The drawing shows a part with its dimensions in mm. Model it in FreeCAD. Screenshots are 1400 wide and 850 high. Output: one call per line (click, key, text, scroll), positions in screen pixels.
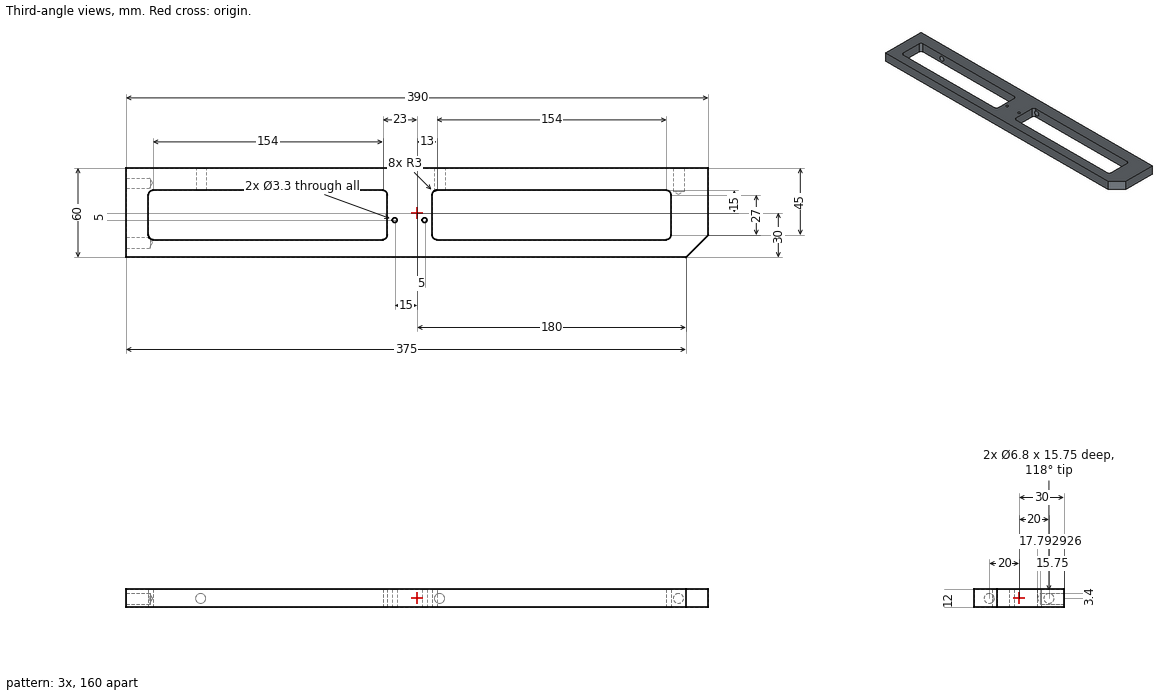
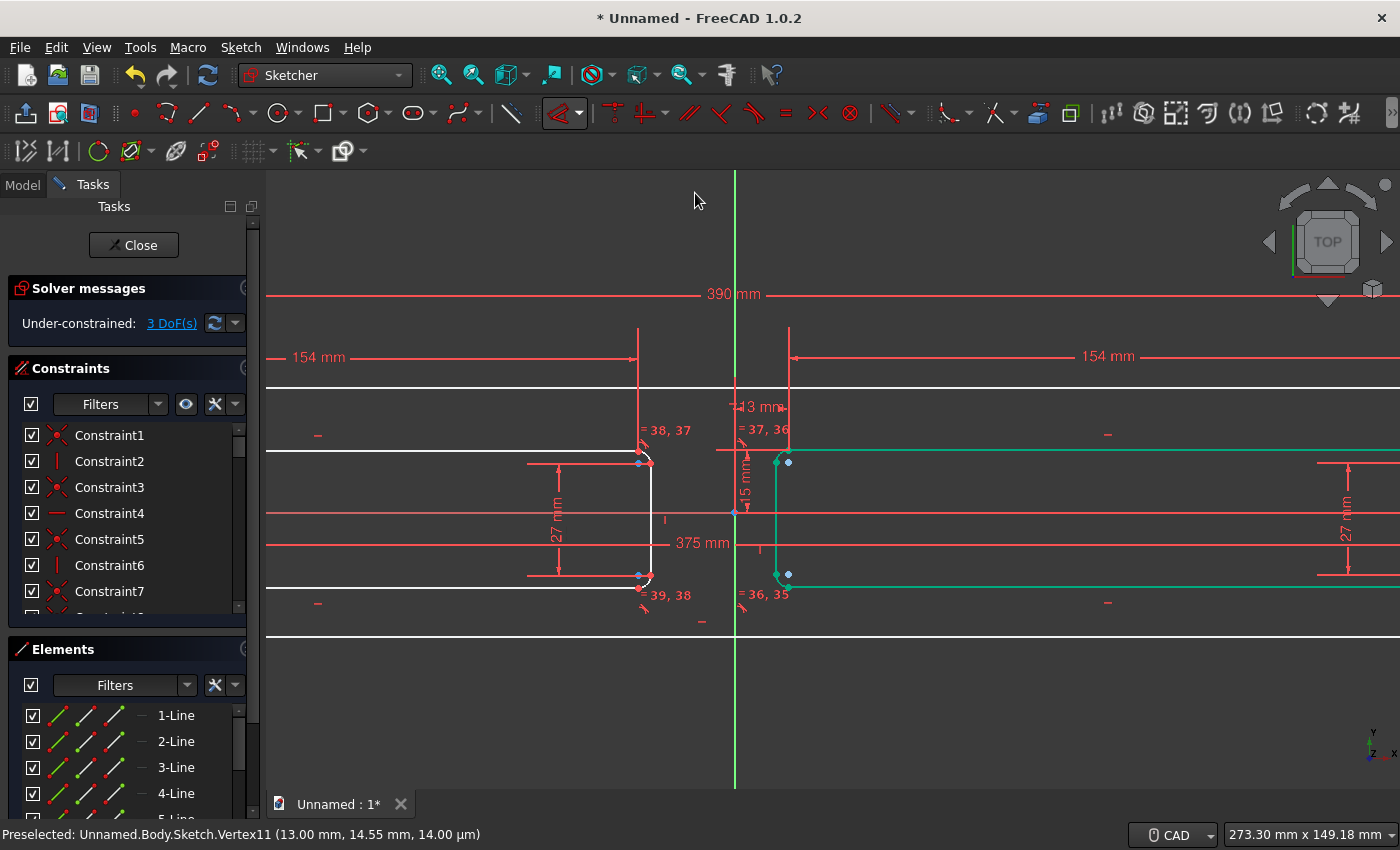
scroll(789, 453, down, 4)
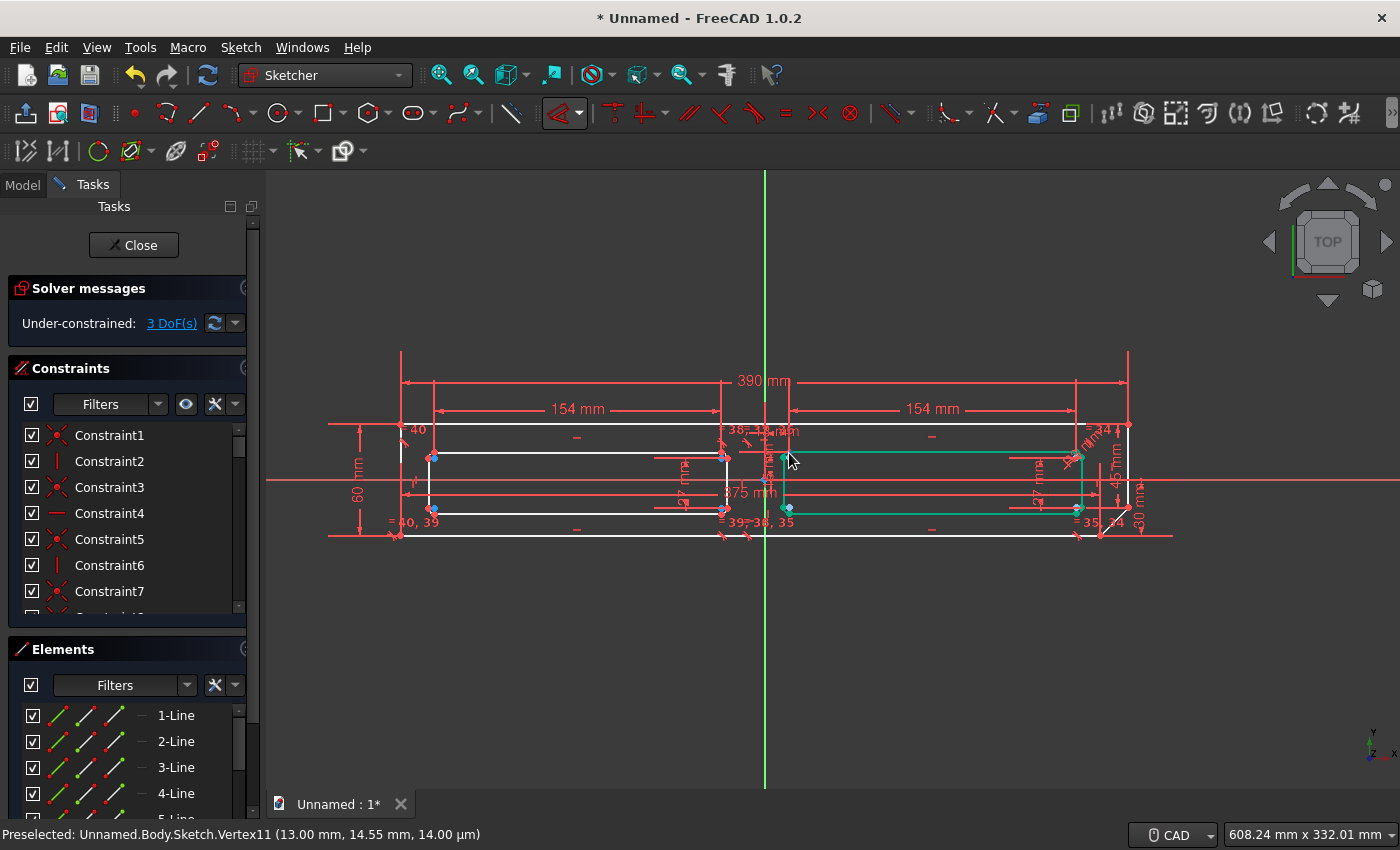
scroll(434, 453, up, 4)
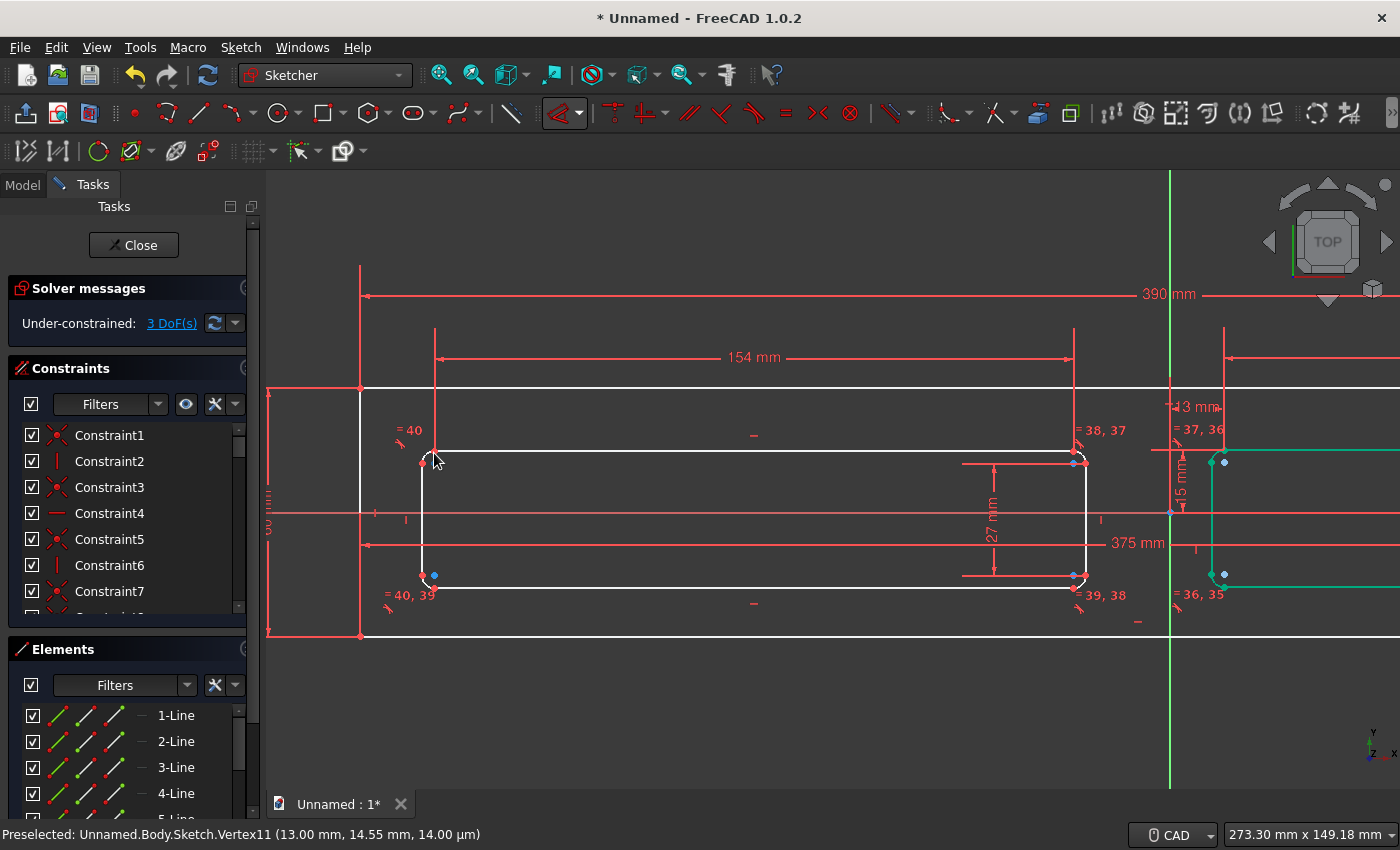
click(435, 451)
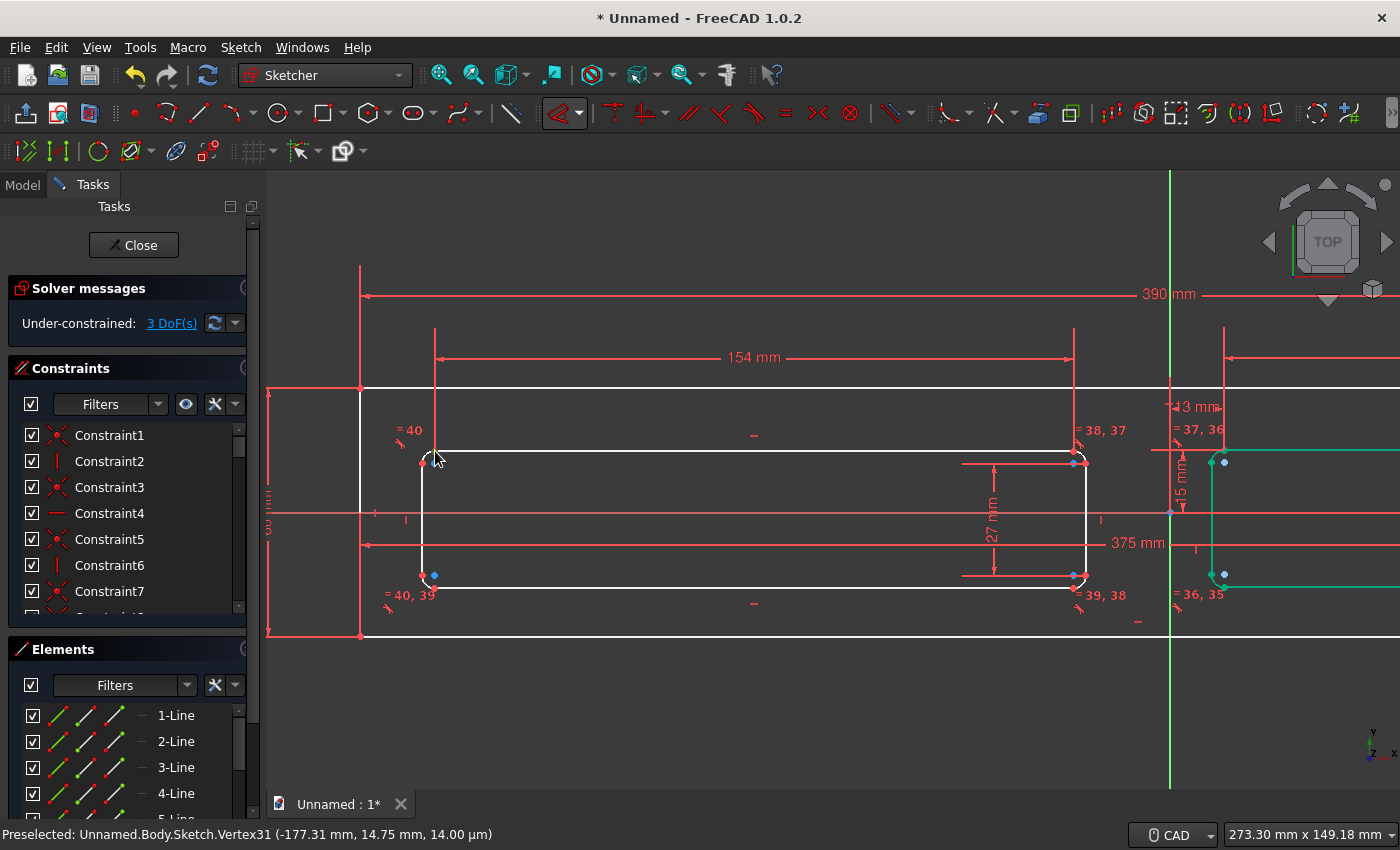
key(i)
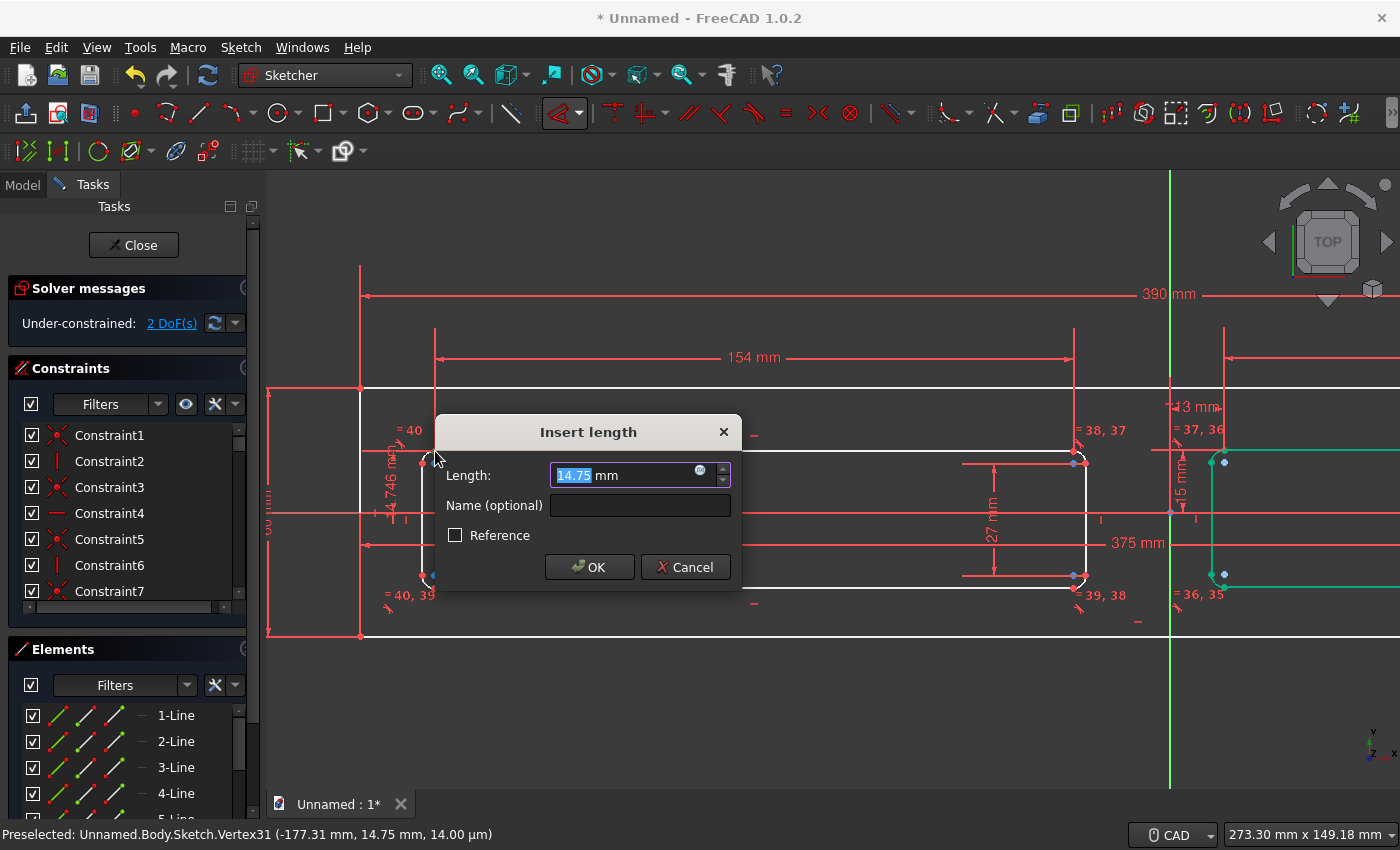
text(15)
key(Return)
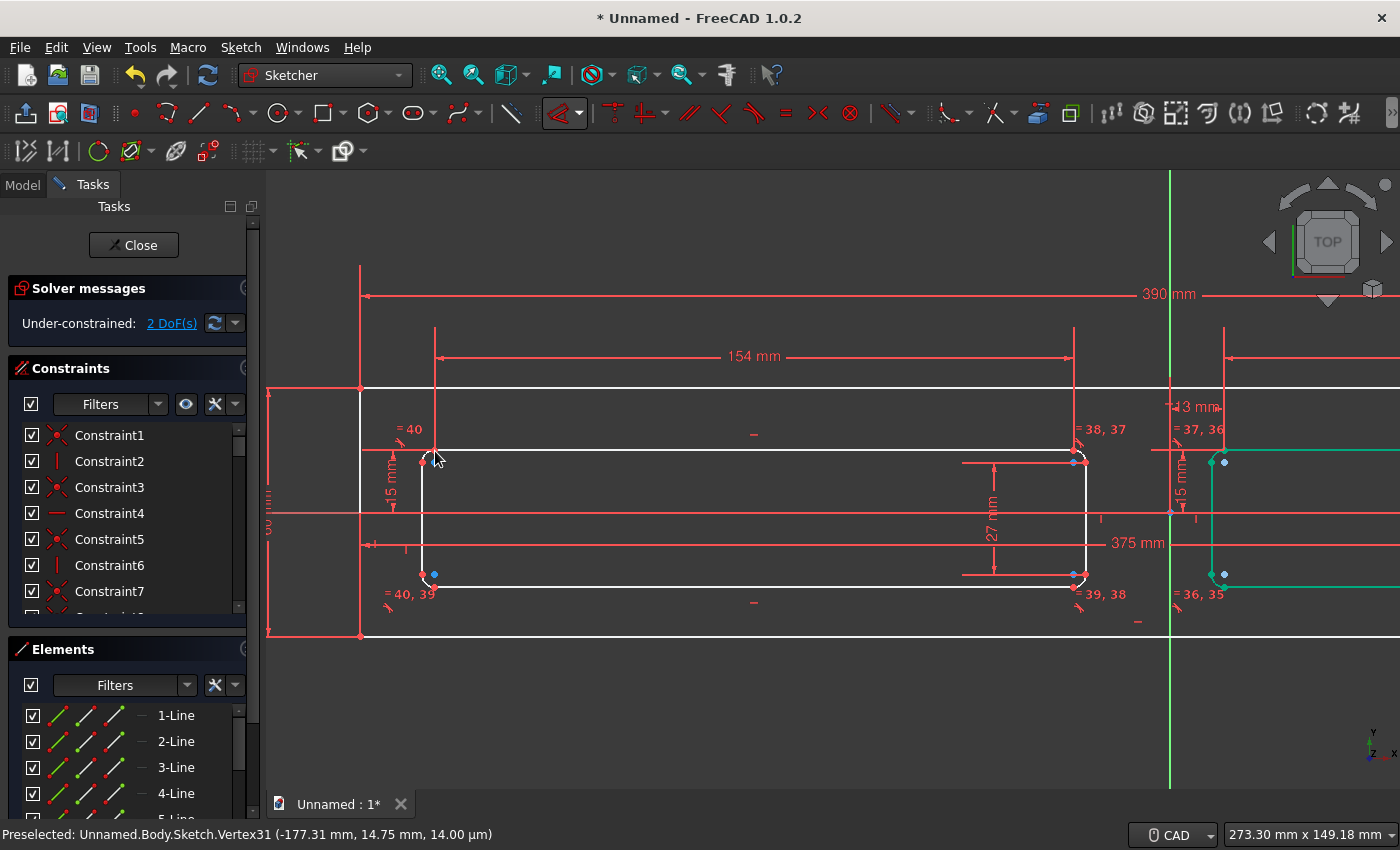
click(1074, 450)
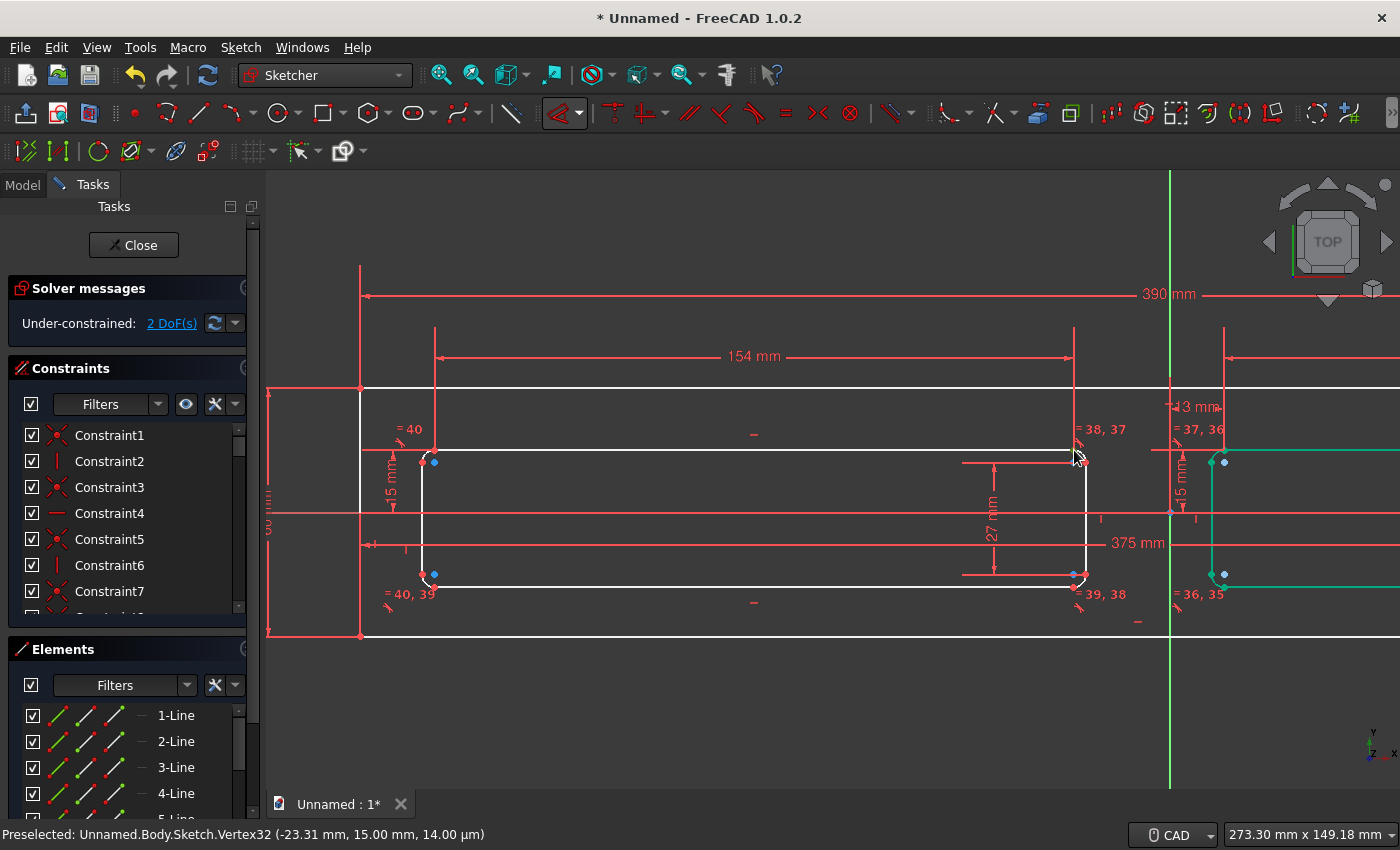
click(582, 114)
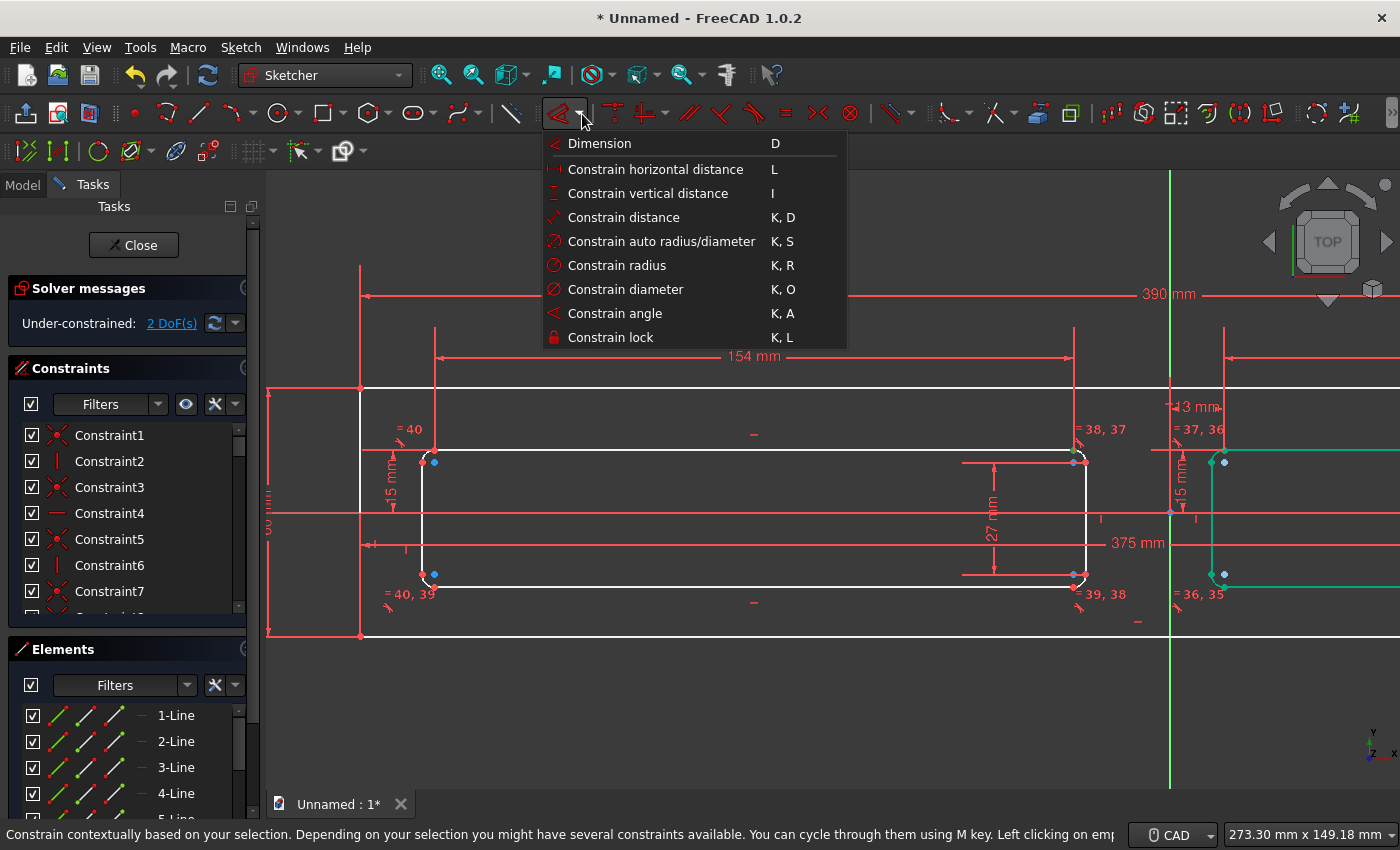
click(695, 169)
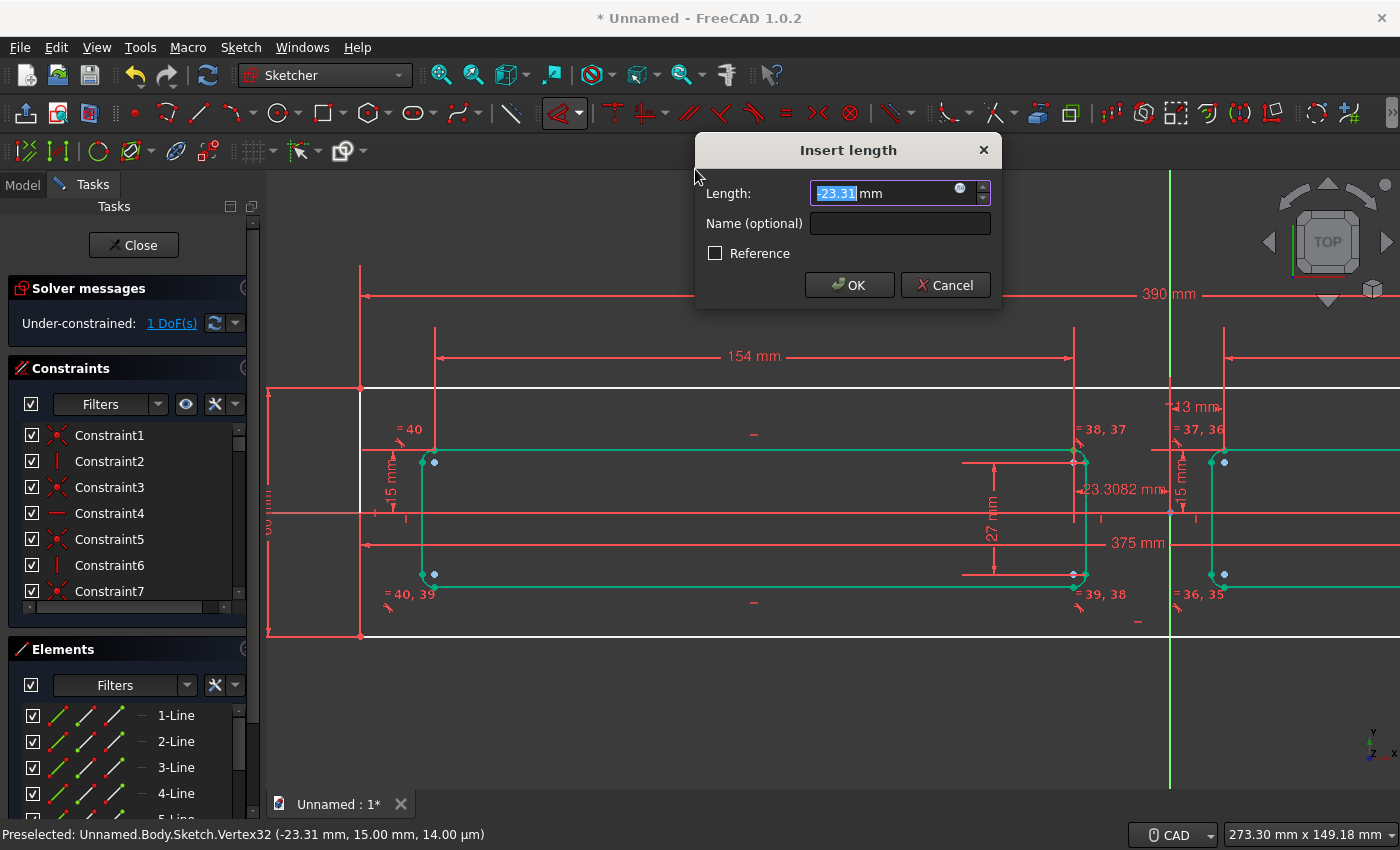
text(-23)
key(Return)